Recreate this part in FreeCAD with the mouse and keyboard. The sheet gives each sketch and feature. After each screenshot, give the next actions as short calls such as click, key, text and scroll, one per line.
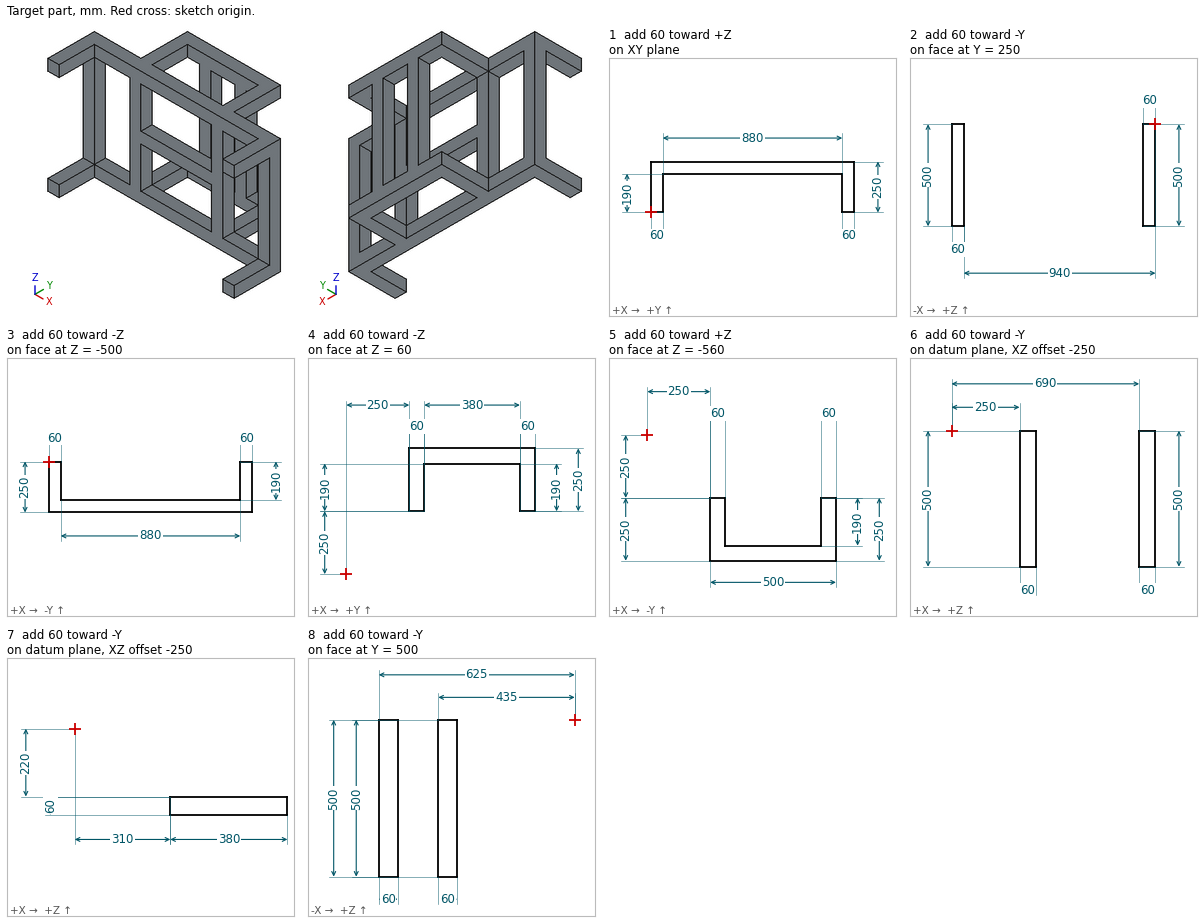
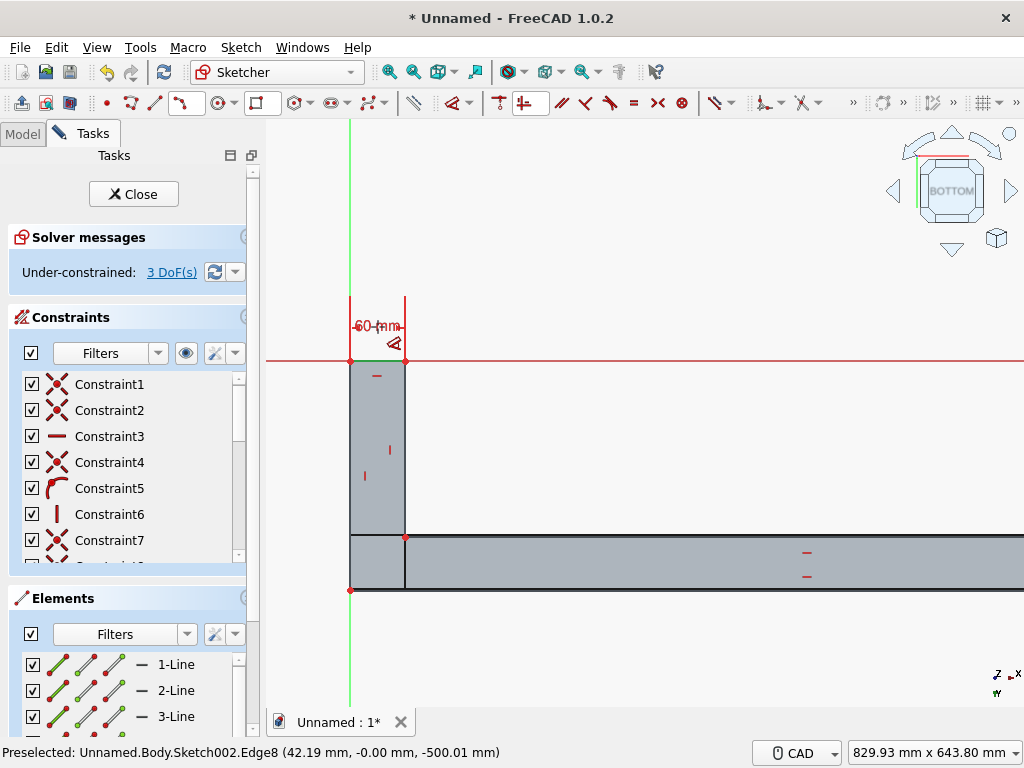
click(350, 430)
click(316, 476)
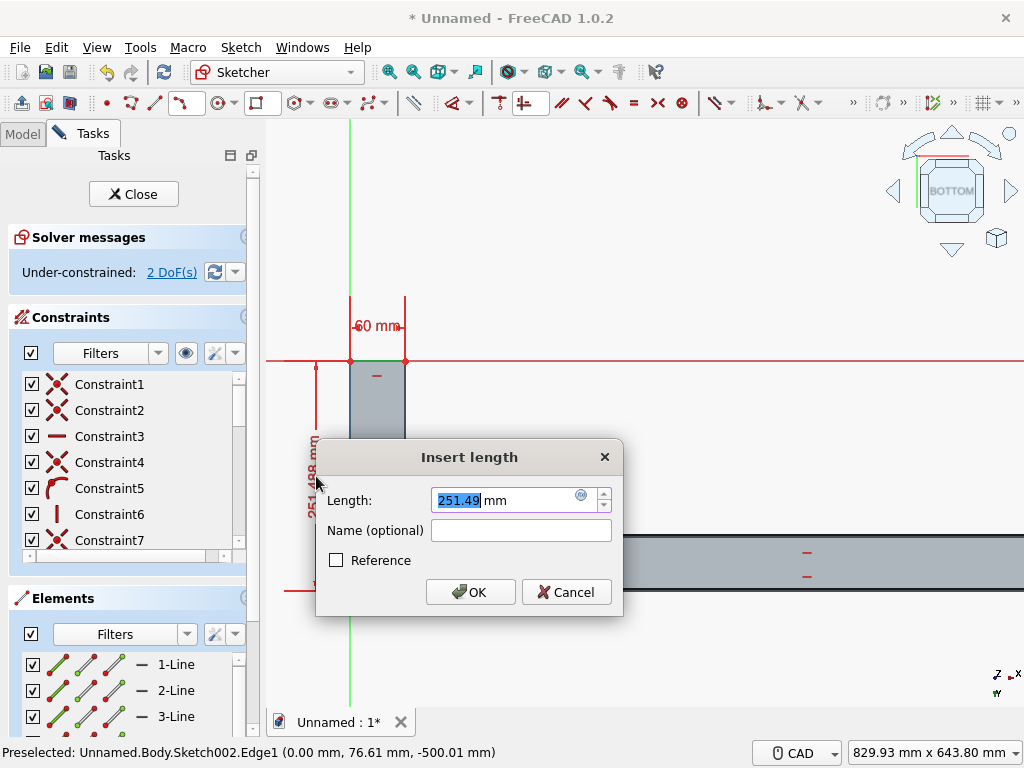
text(250)
key(Return)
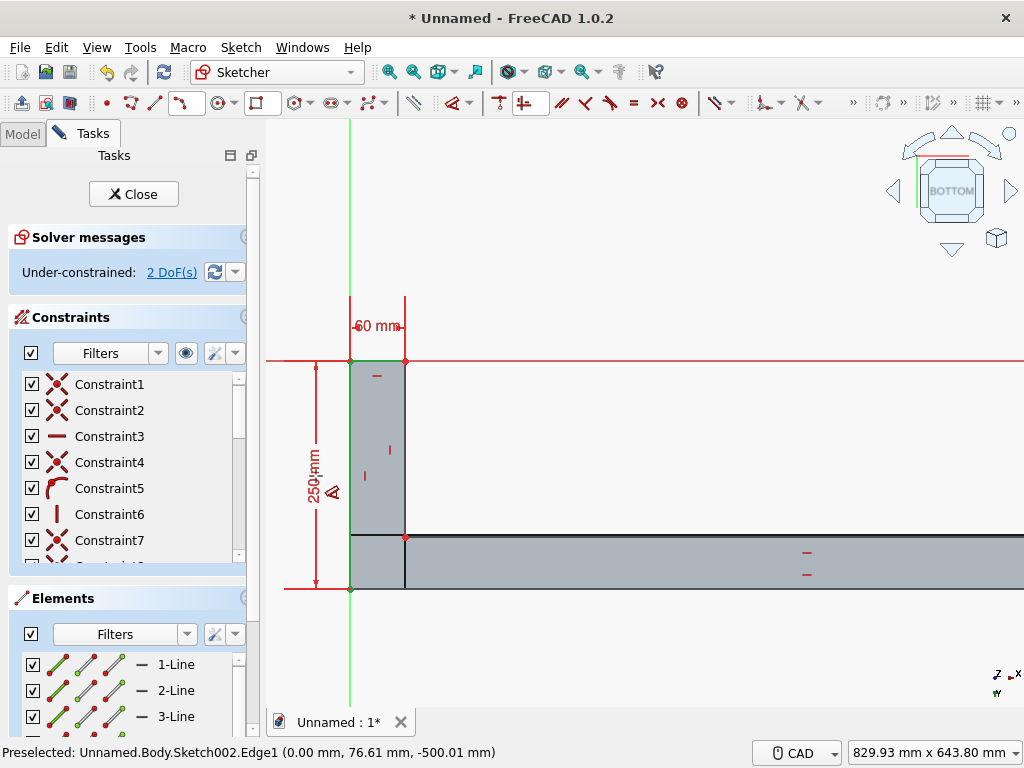
scroll(388, 362, down, 4)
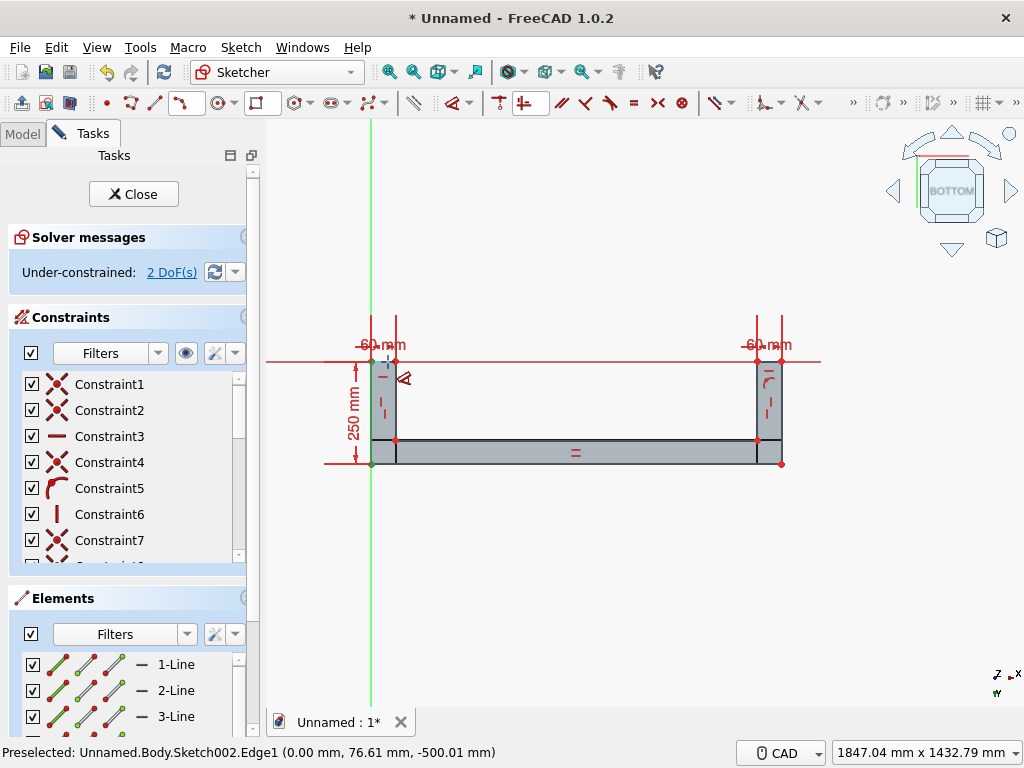
click(757, 386)
click(723, 401)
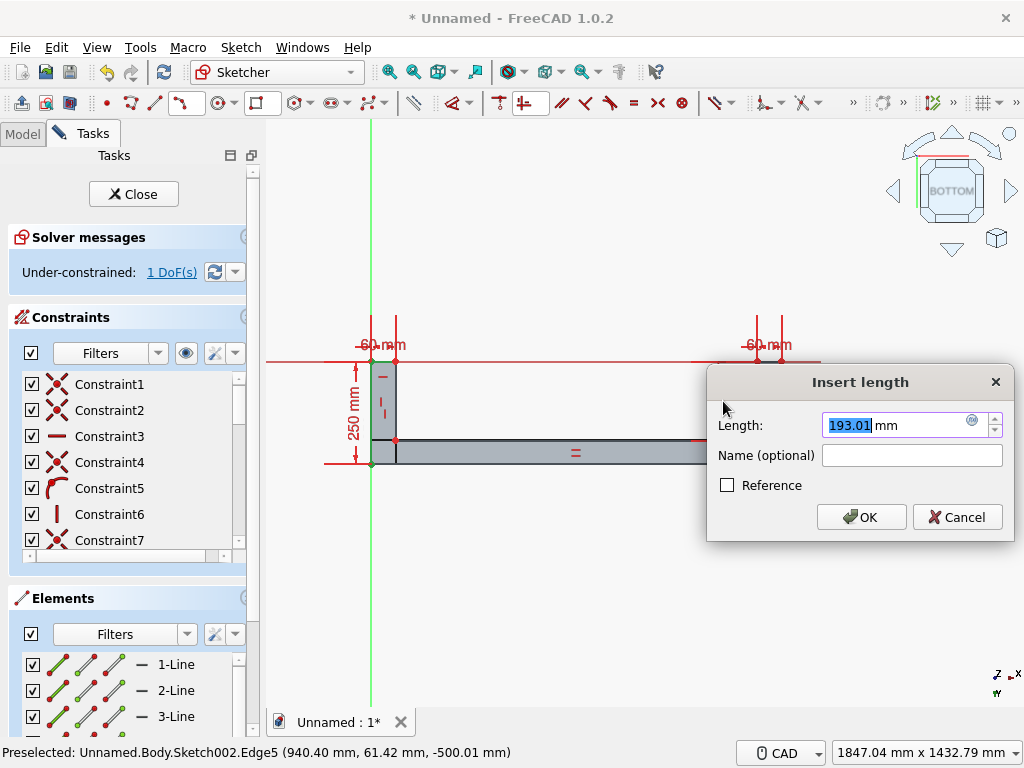
text(190)
key(Return)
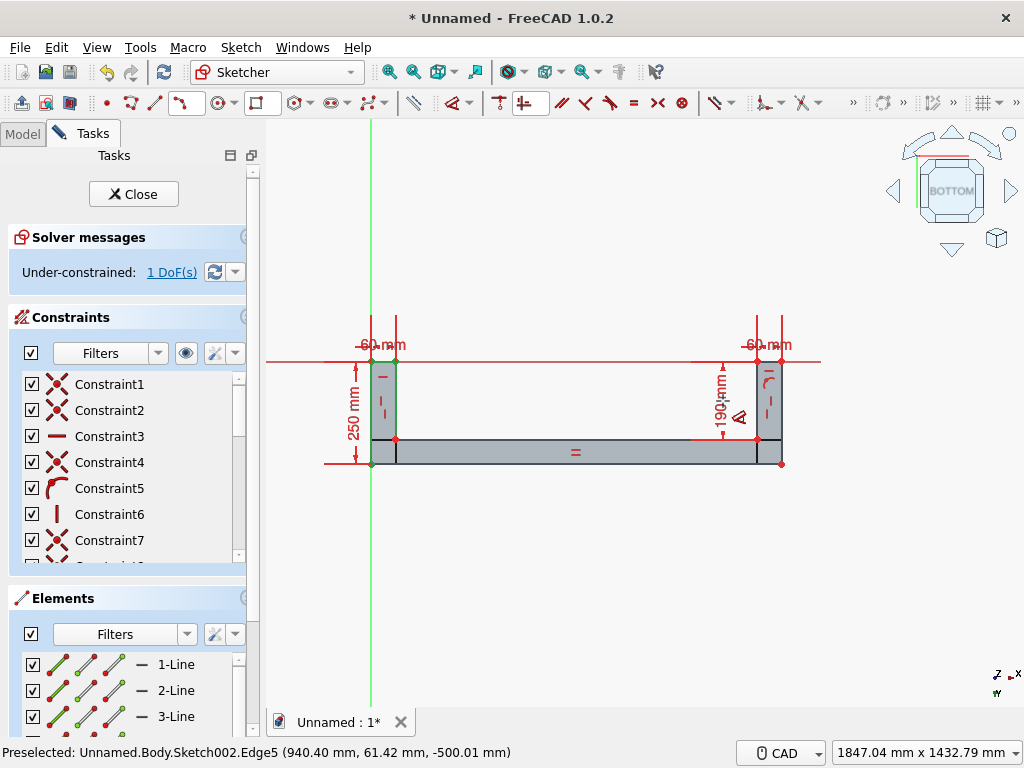
click(649, 440)
click(577, 406)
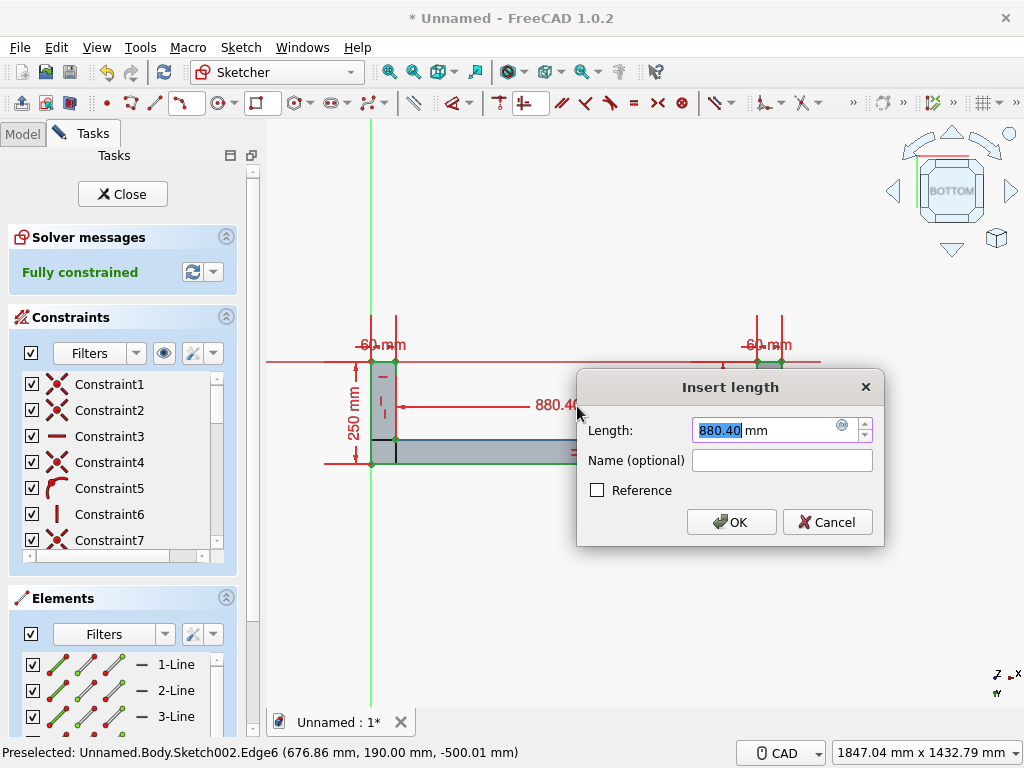
text(880)
key(Return)
key(Escape)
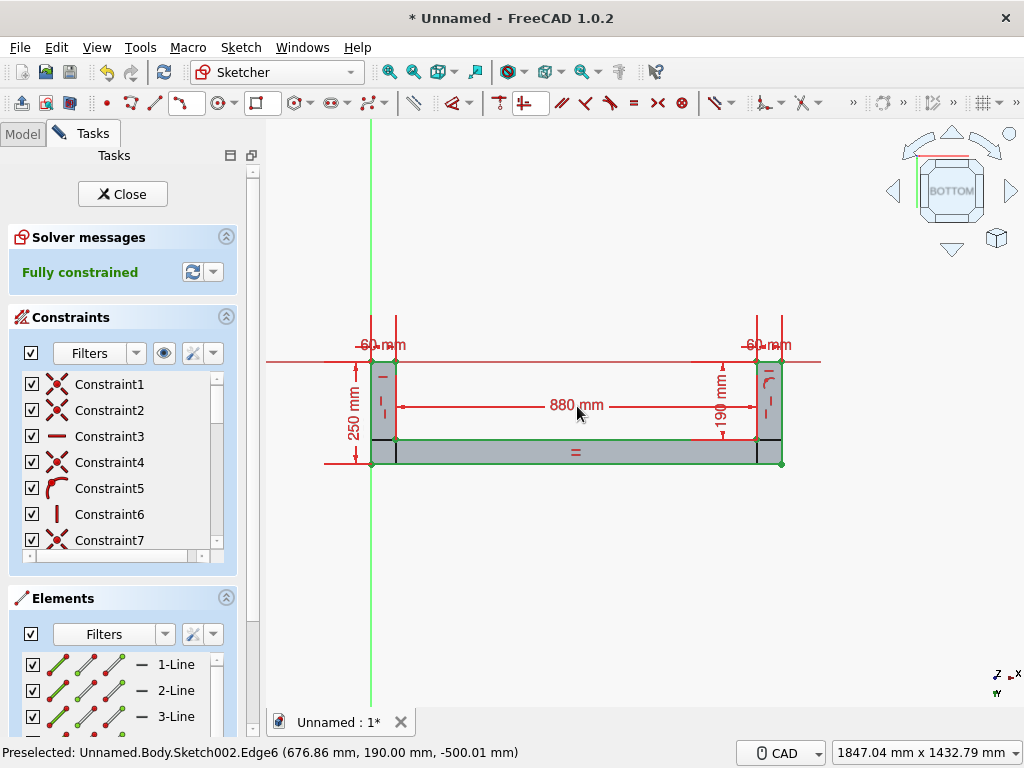
click(123, 194)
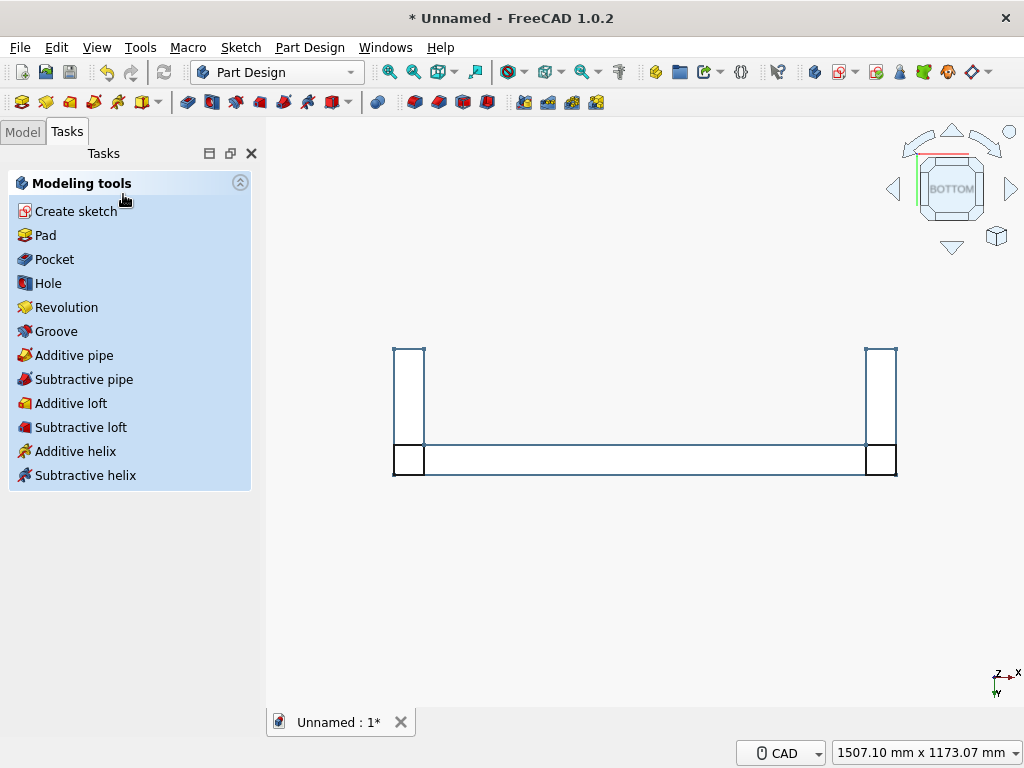
click(22, 102)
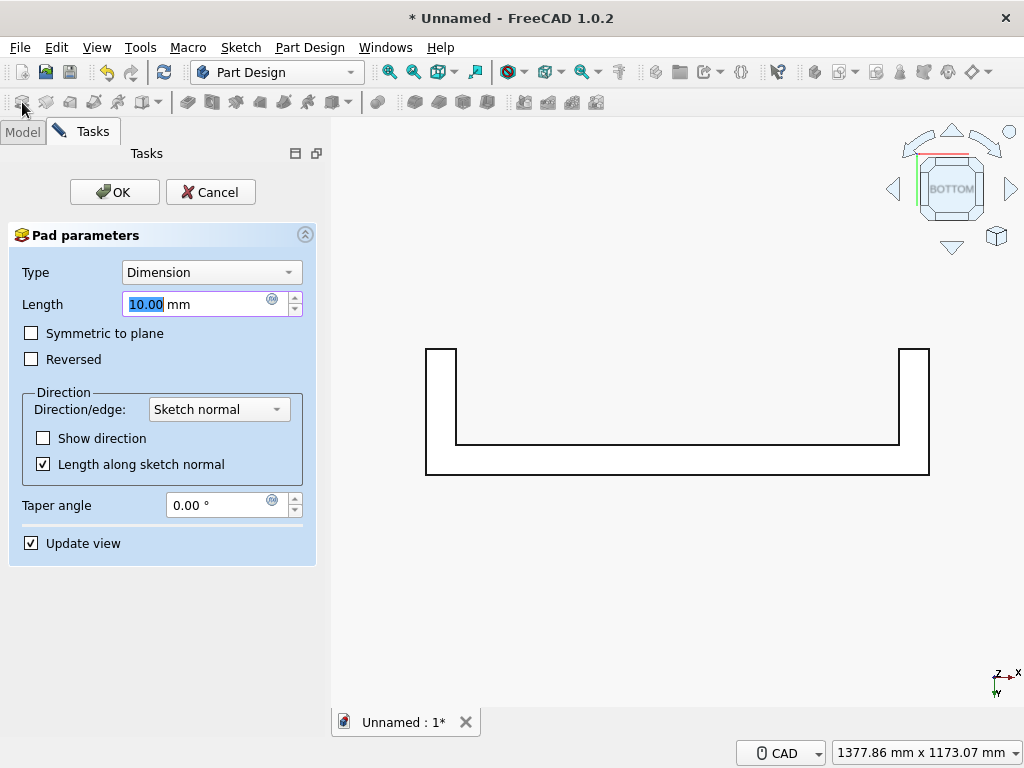
text(60)
key(Tab)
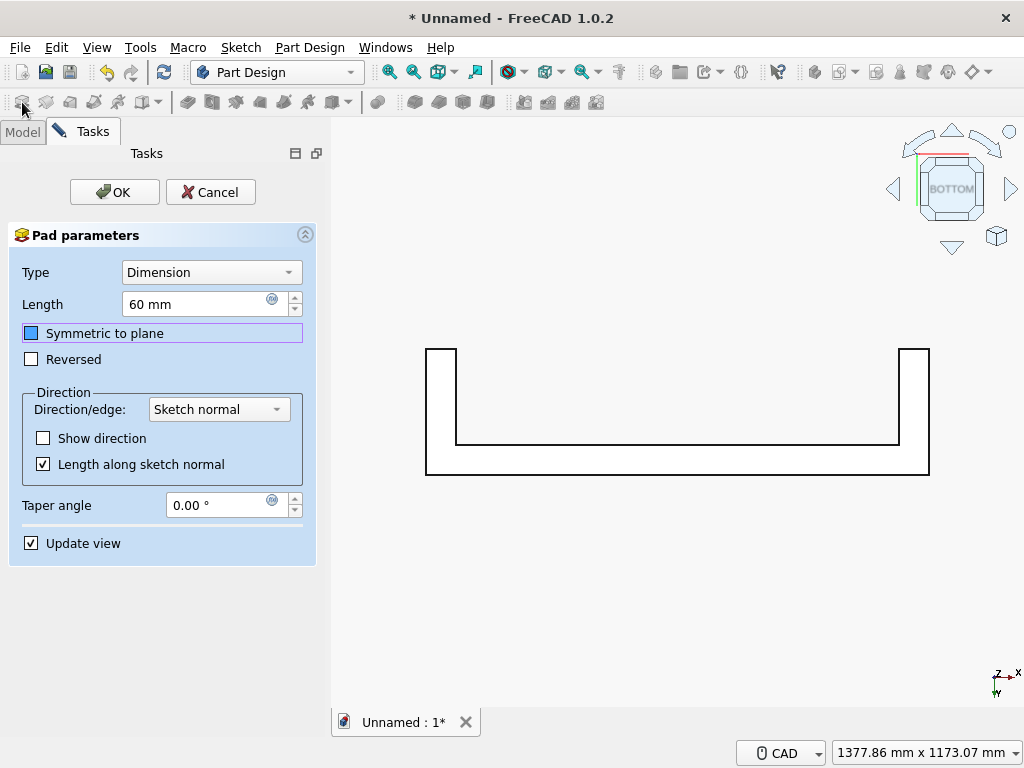
click(115, 192)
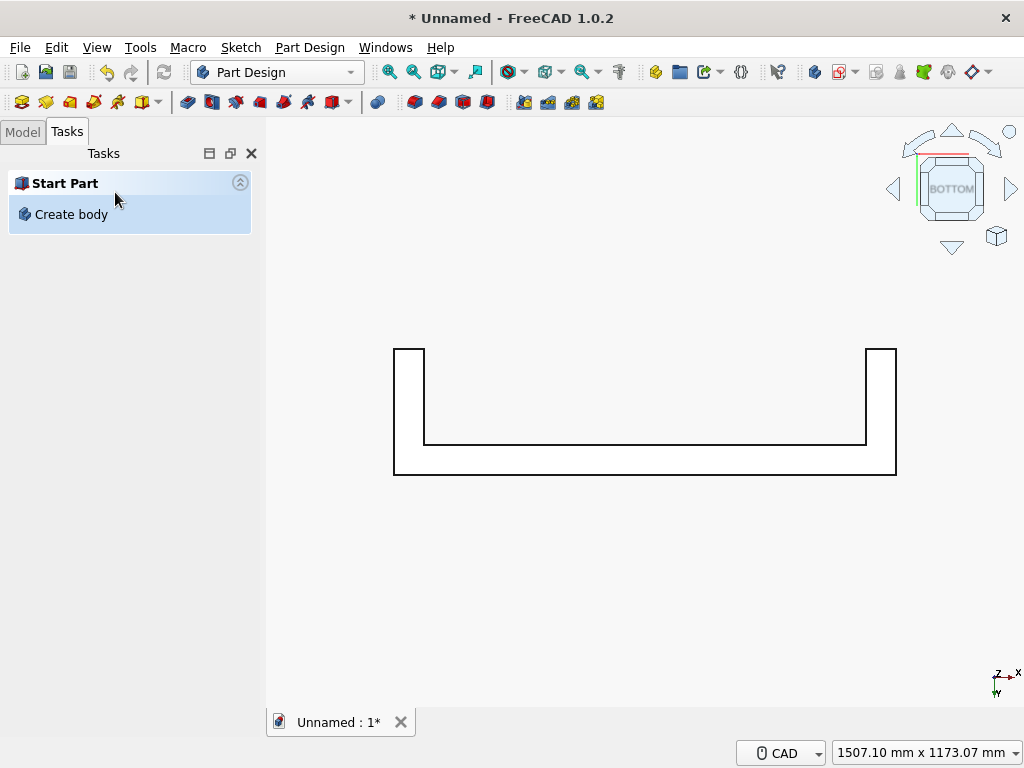
key(0)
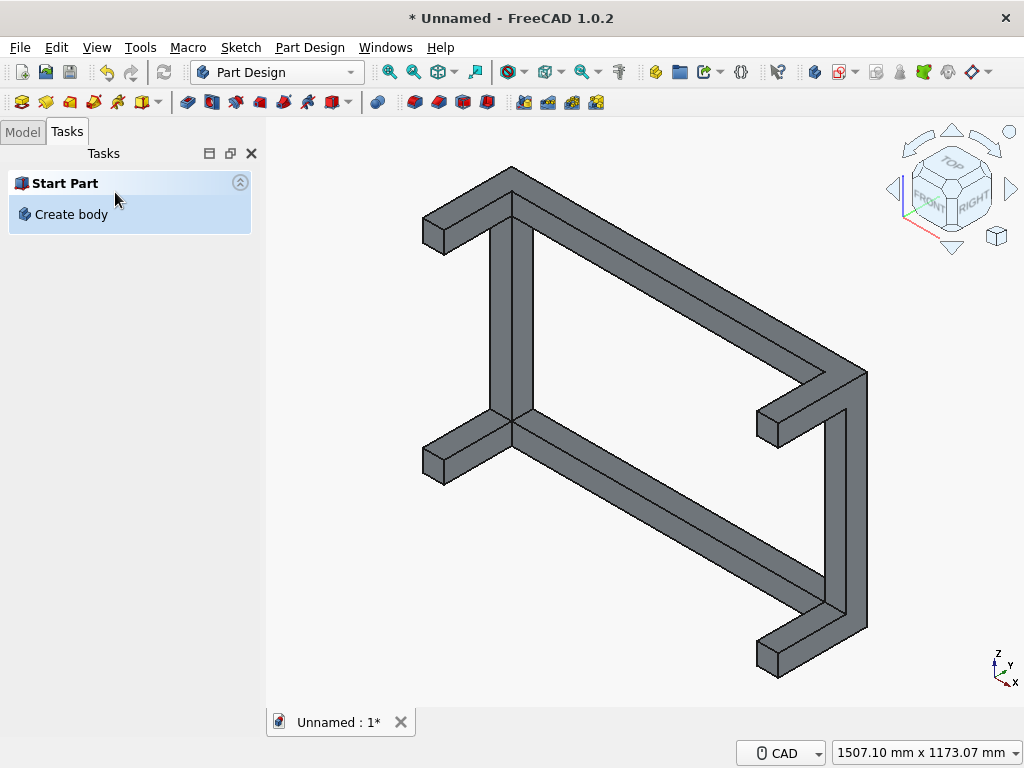
click(836, 360)